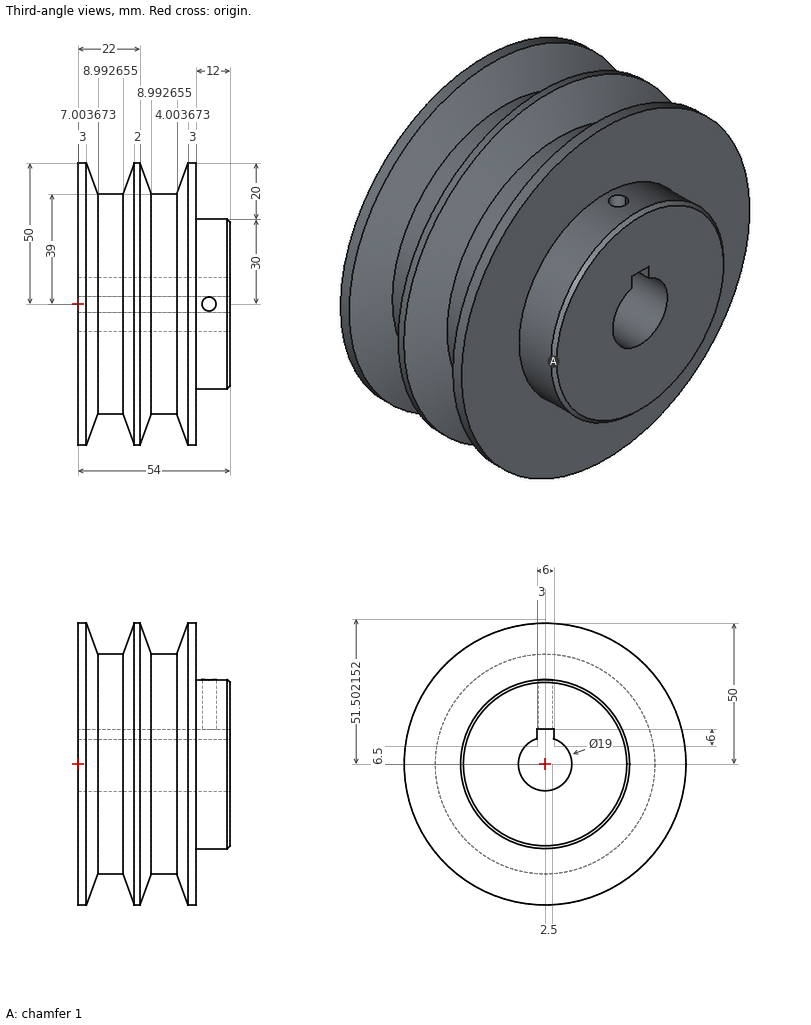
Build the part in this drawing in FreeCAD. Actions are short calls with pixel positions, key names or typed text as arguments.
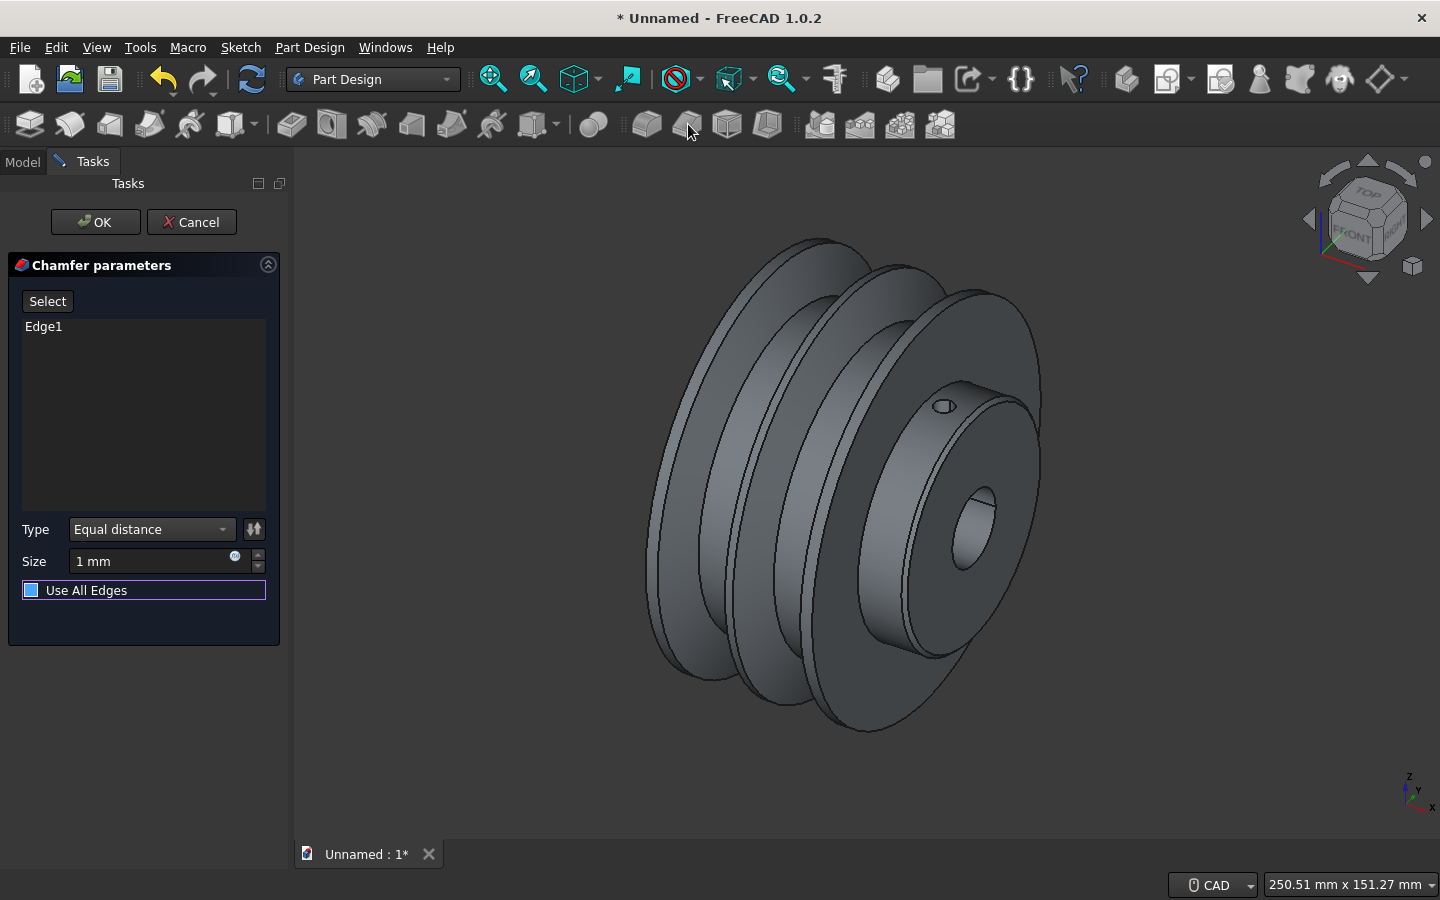
click(96, 222)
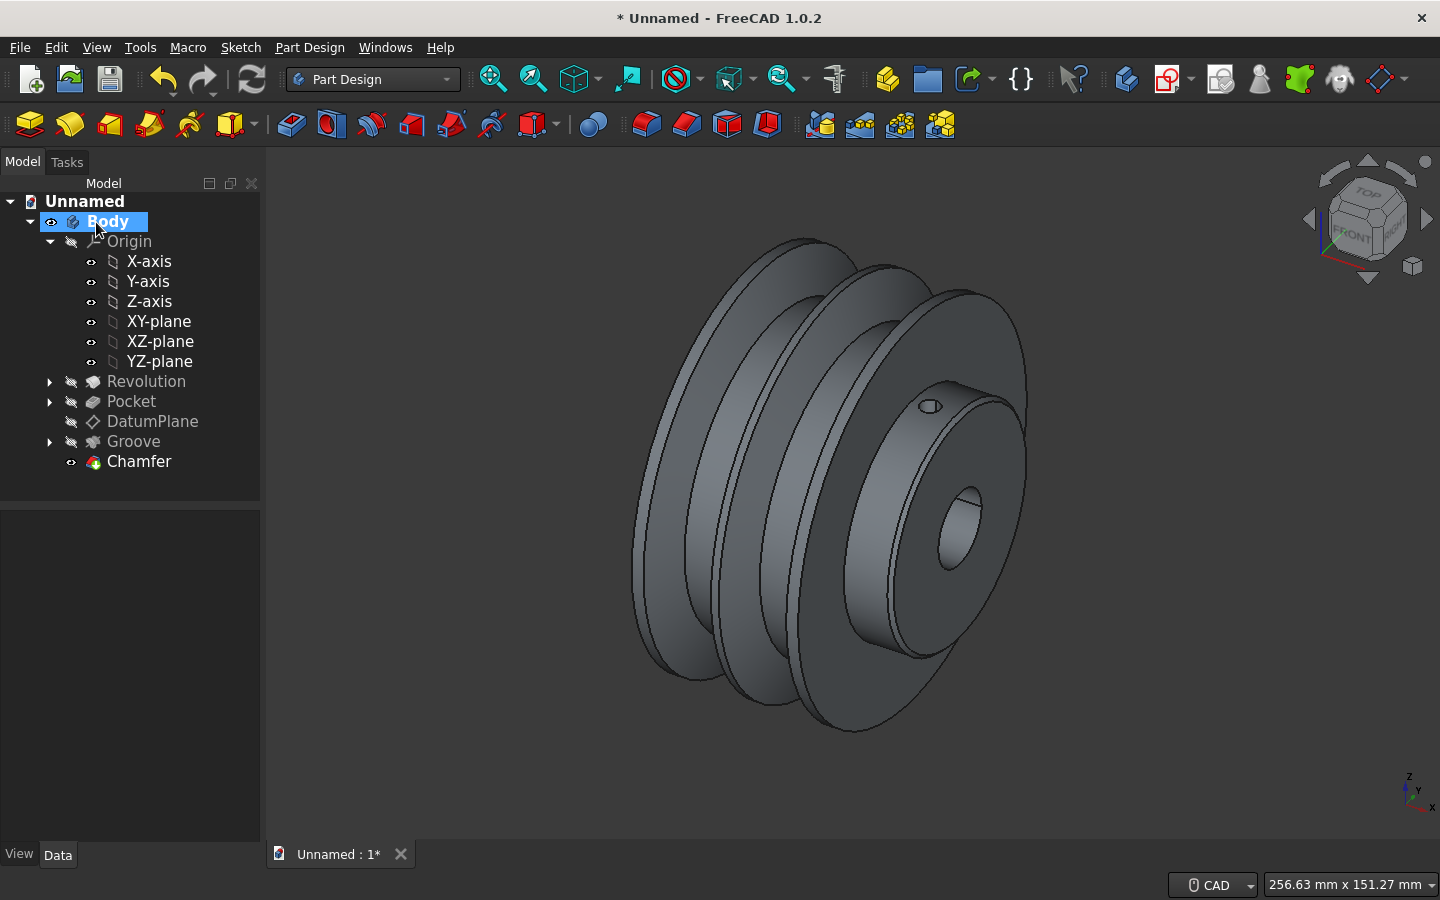
click(998, 521)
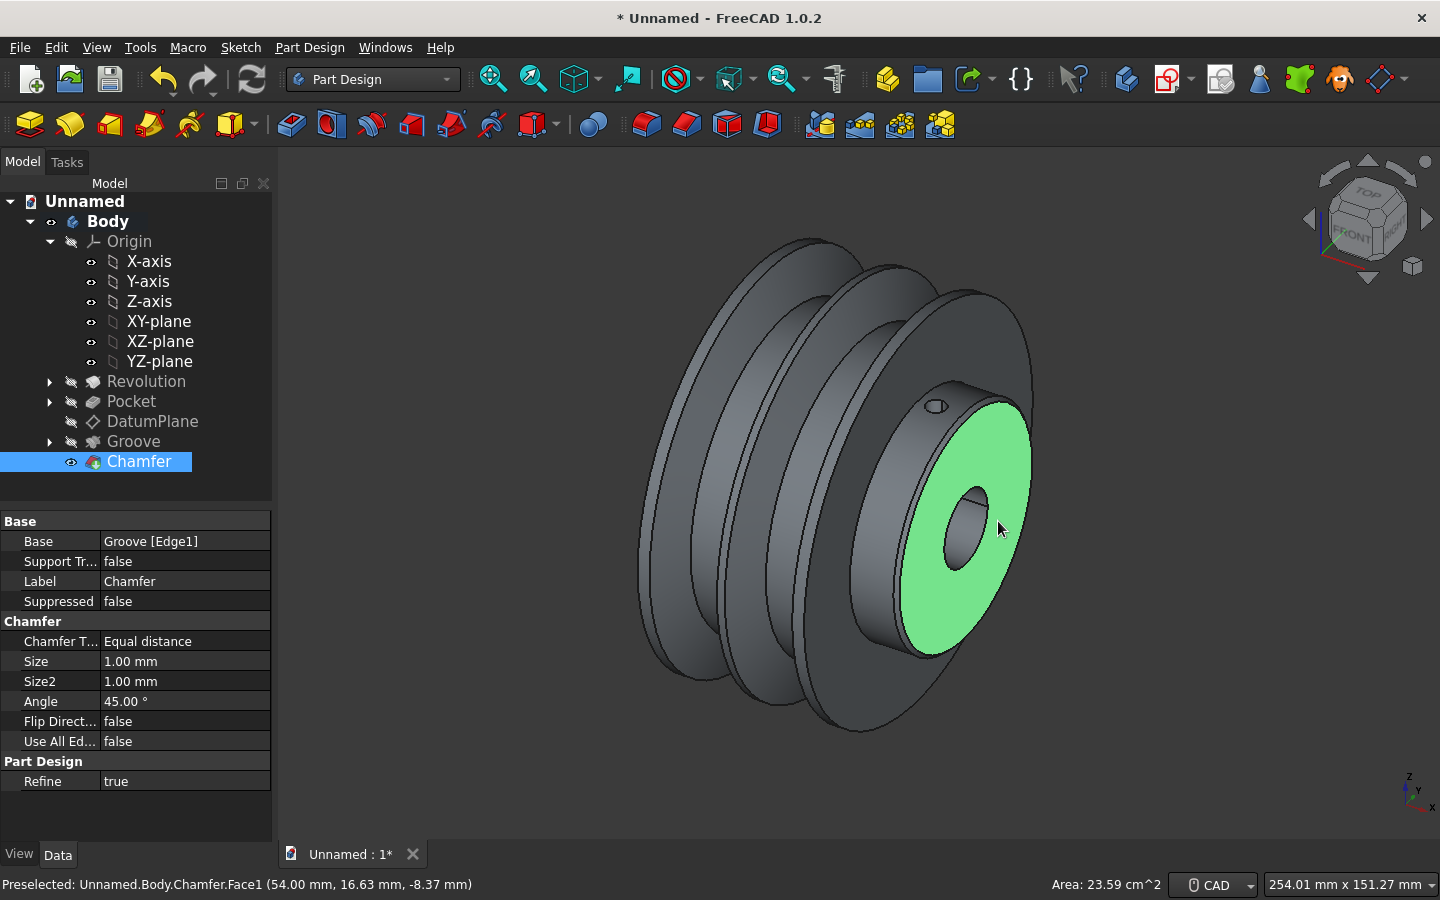
click(1168, 80)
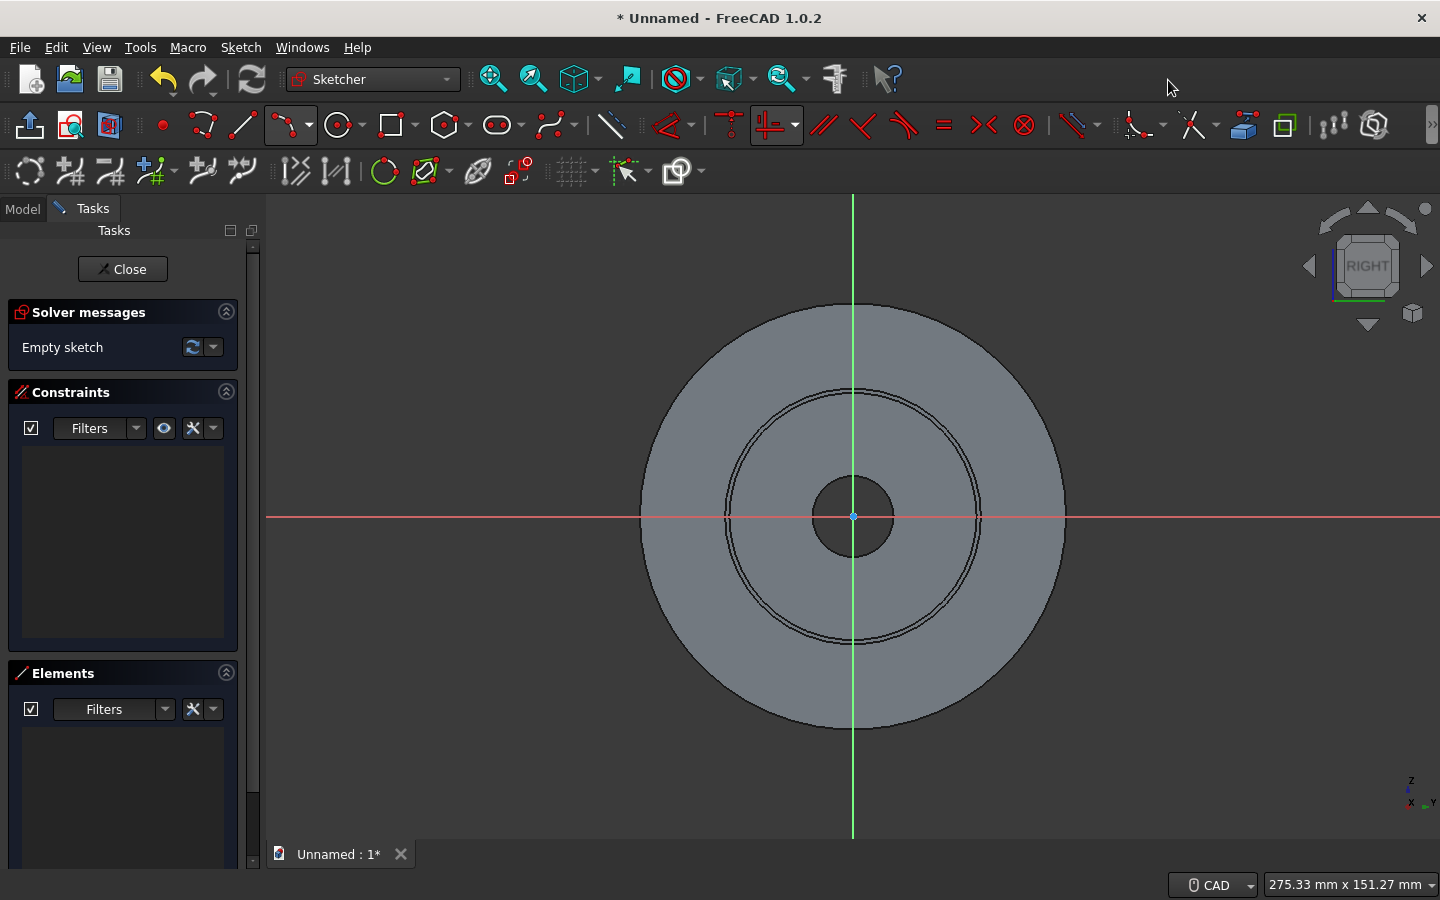
scroll(864, 486, up, 10)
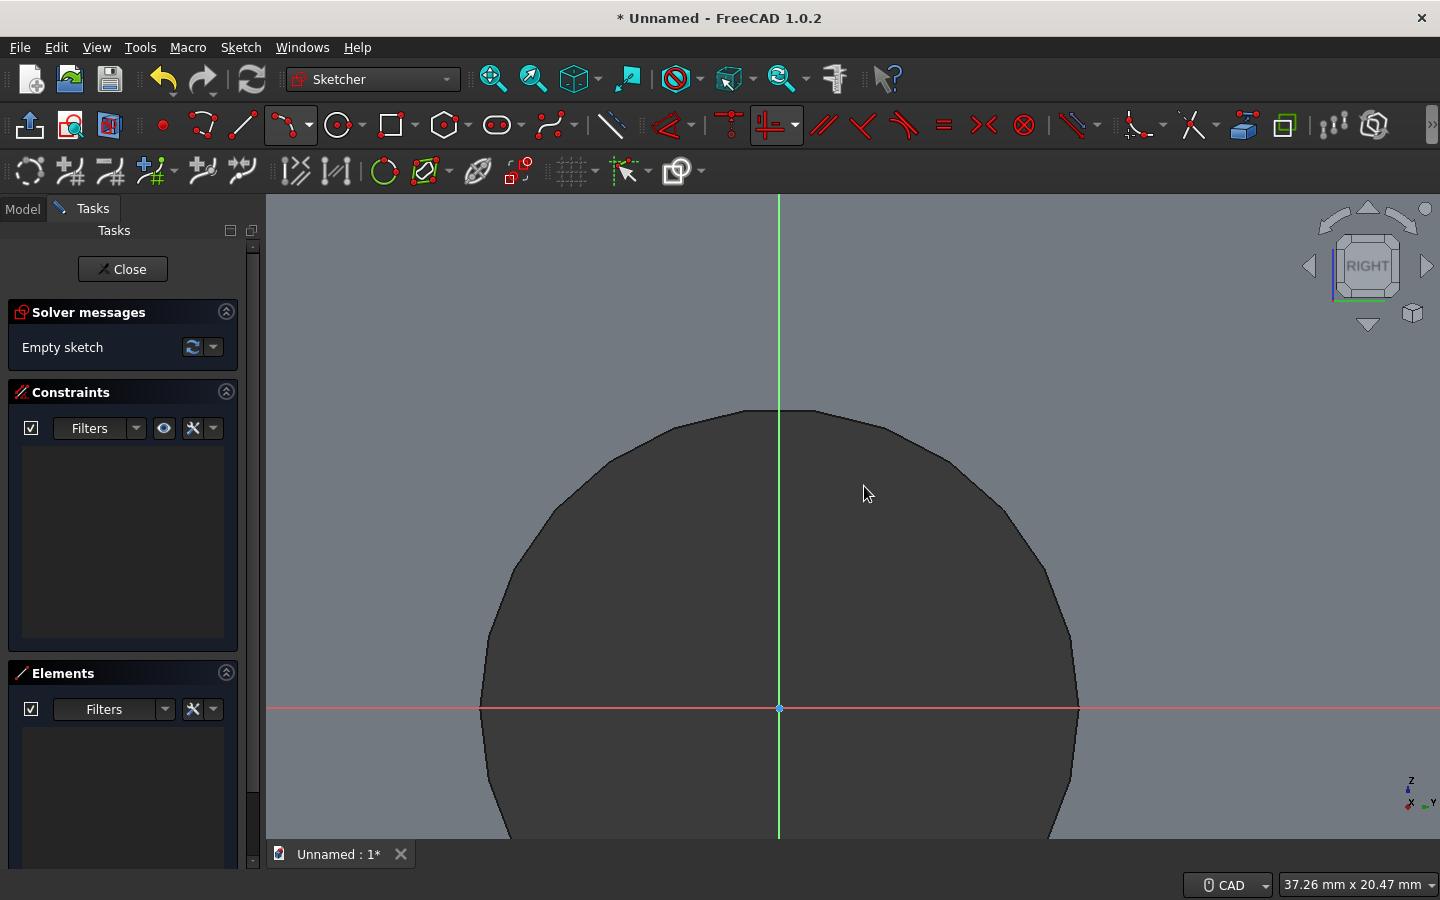
click(392, 126)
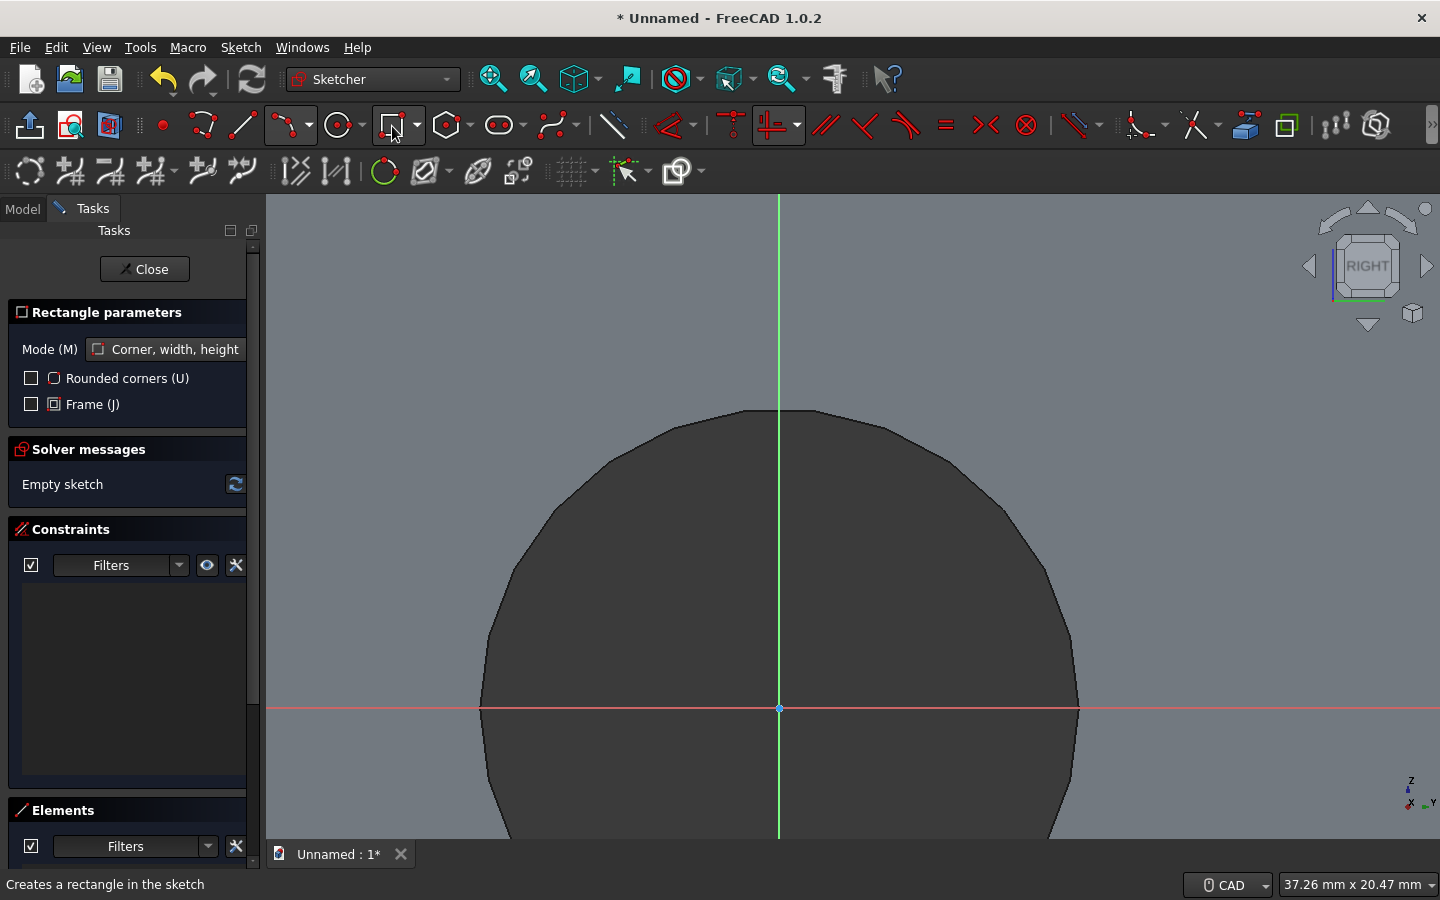
click(685, 315)
move(874, 504)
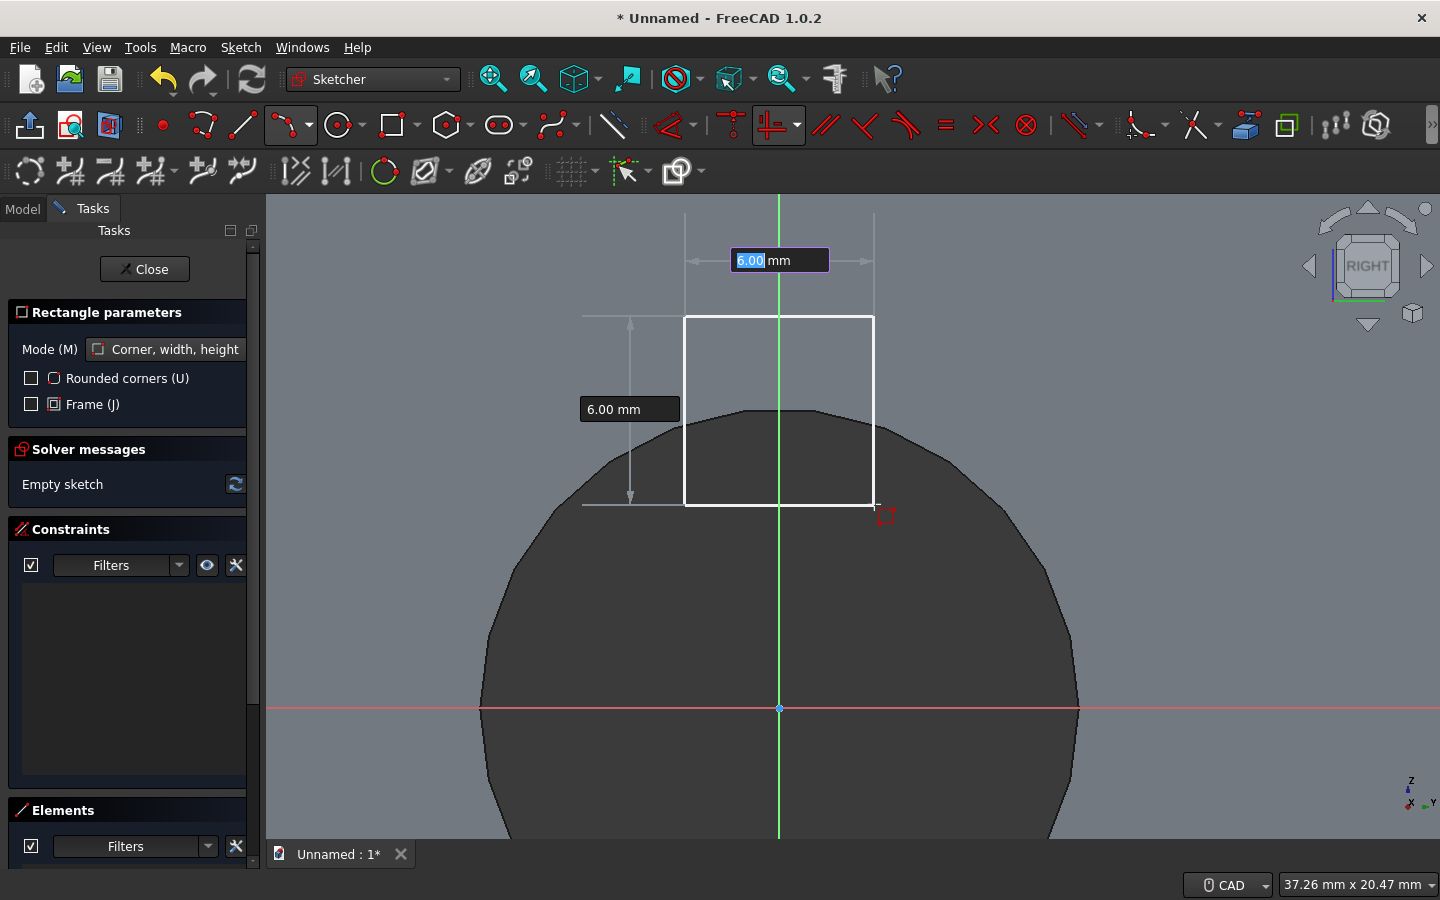
text(6)
key(Tab)
text(6)
key(Return)
key(Escape)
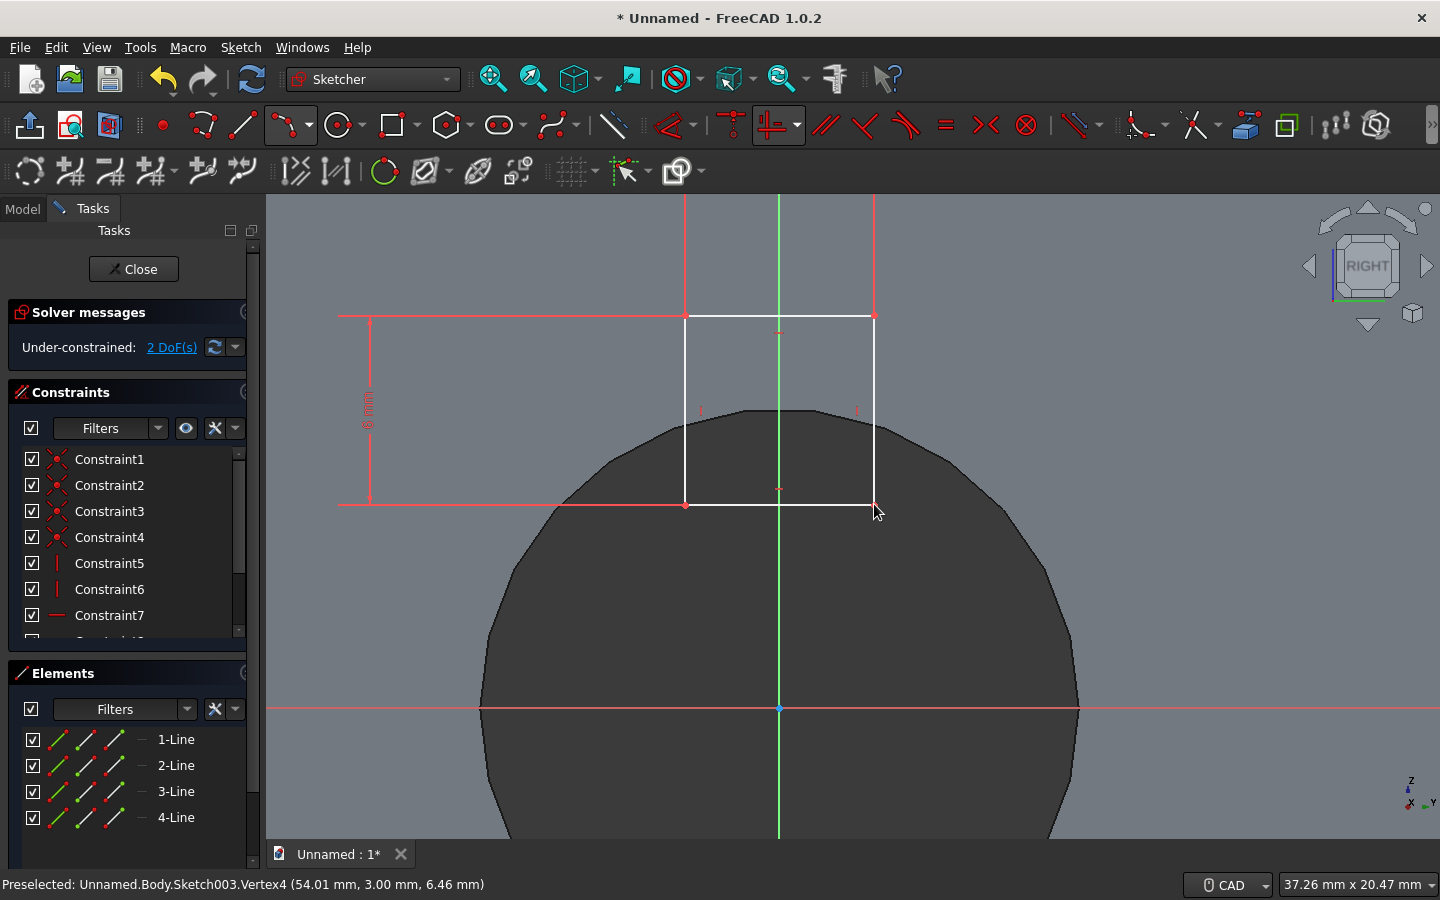
click(668, 126)